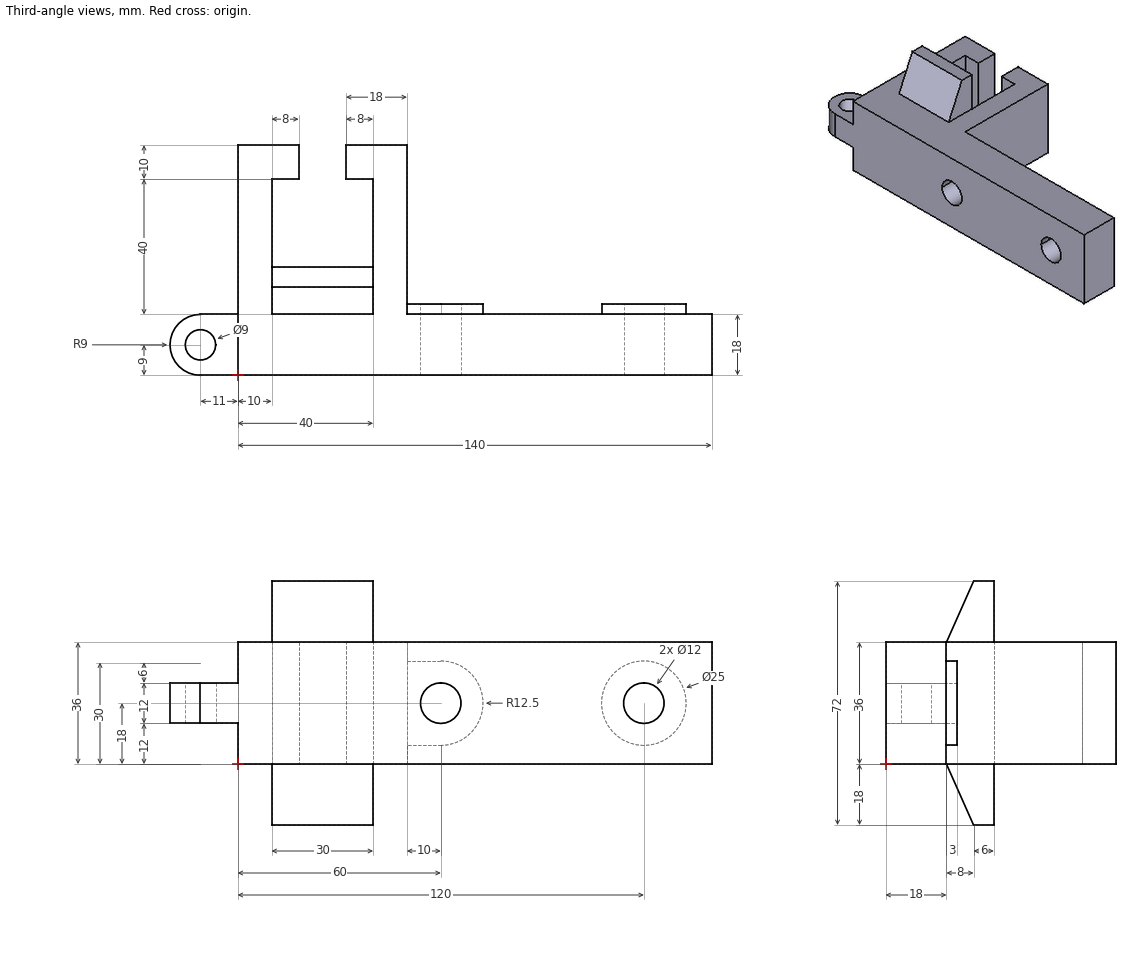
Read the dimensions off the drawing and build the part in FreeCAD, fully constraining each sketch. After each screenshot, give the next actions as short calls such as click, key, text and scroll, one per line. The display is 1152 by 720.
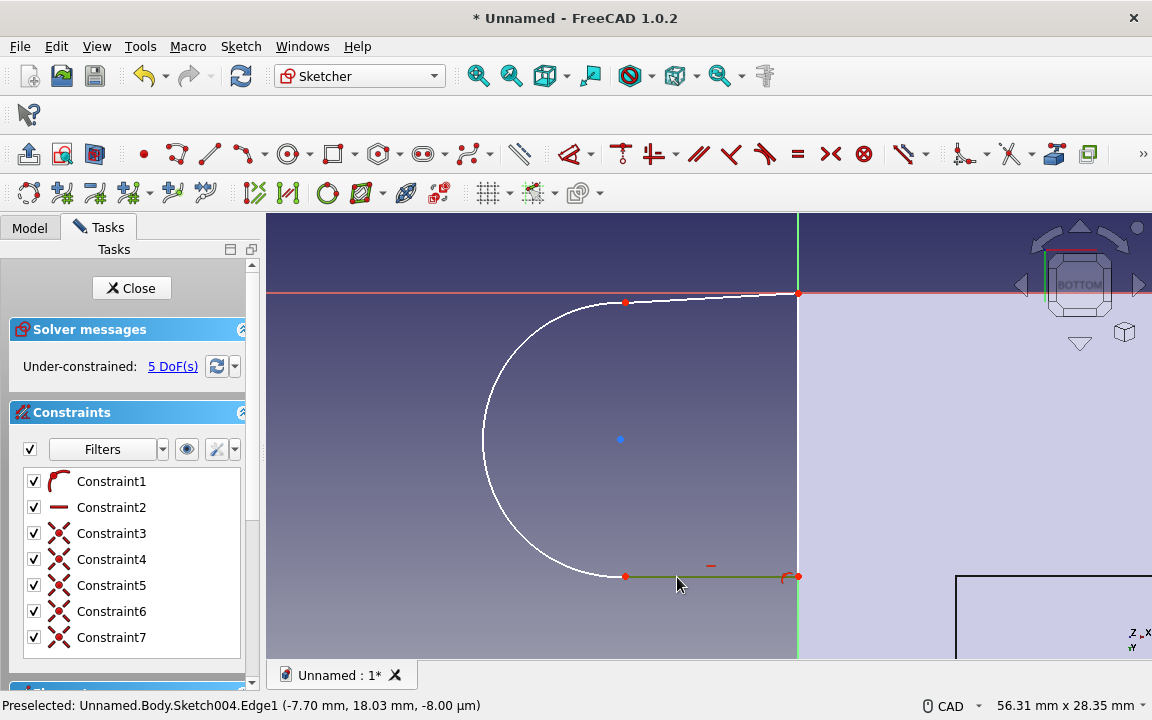
click(510, 358)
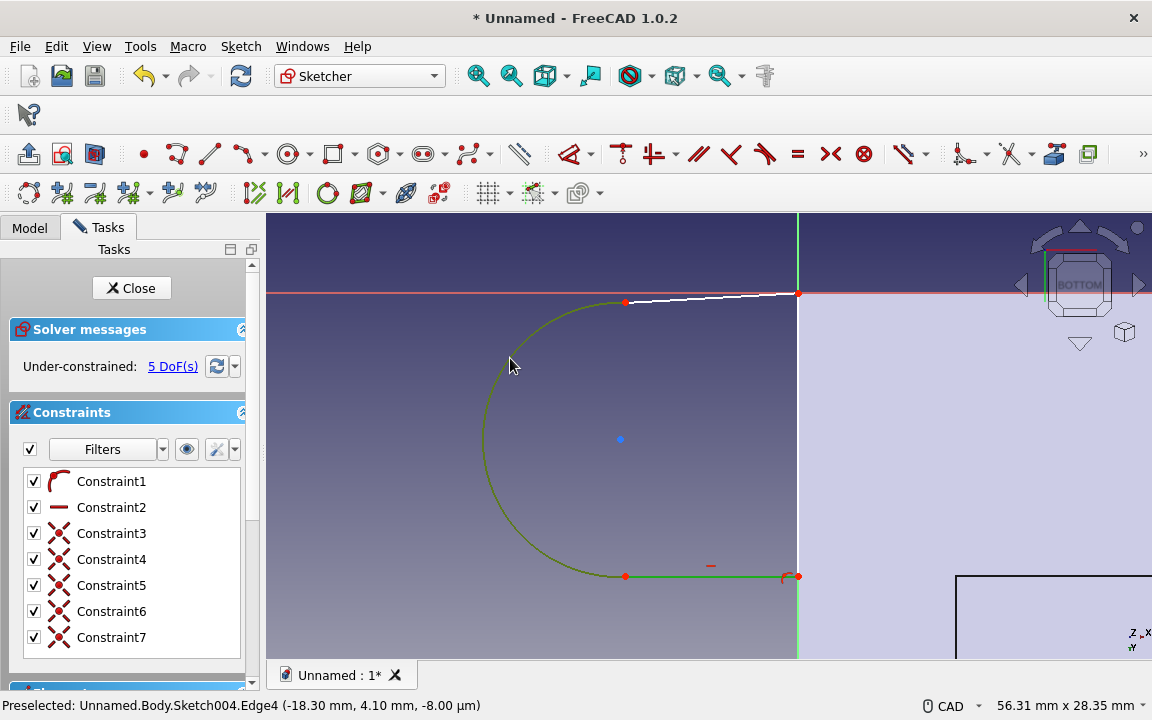
click(765, 154)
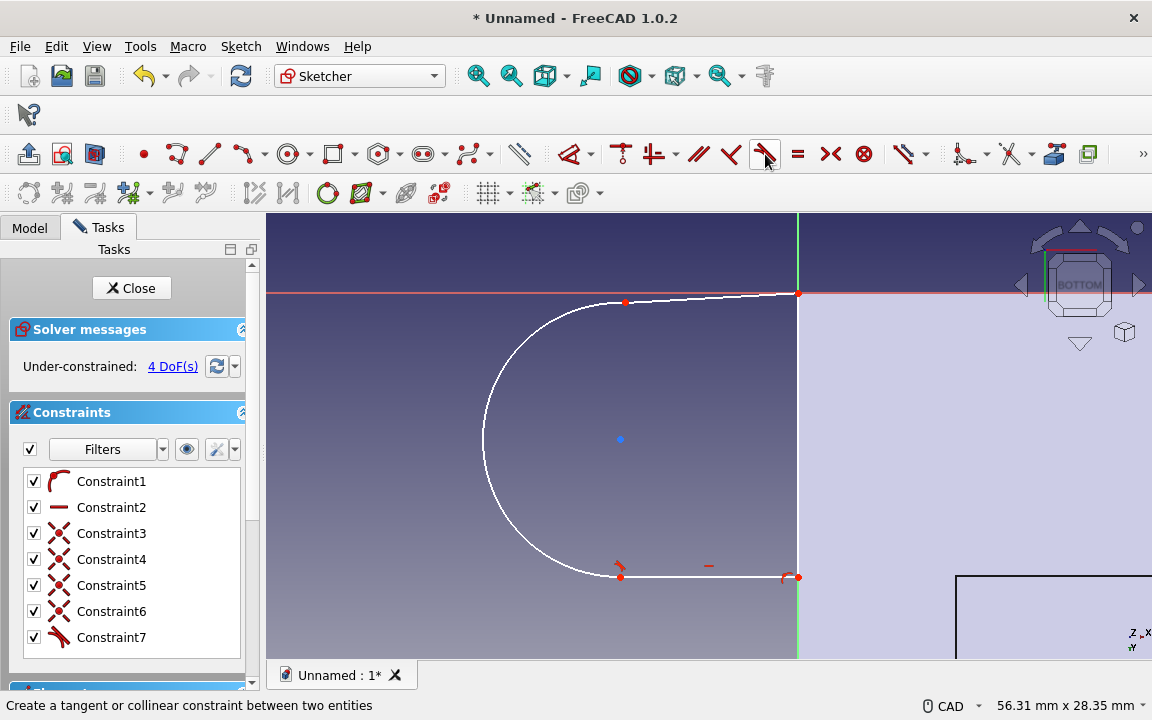
click(746, 296)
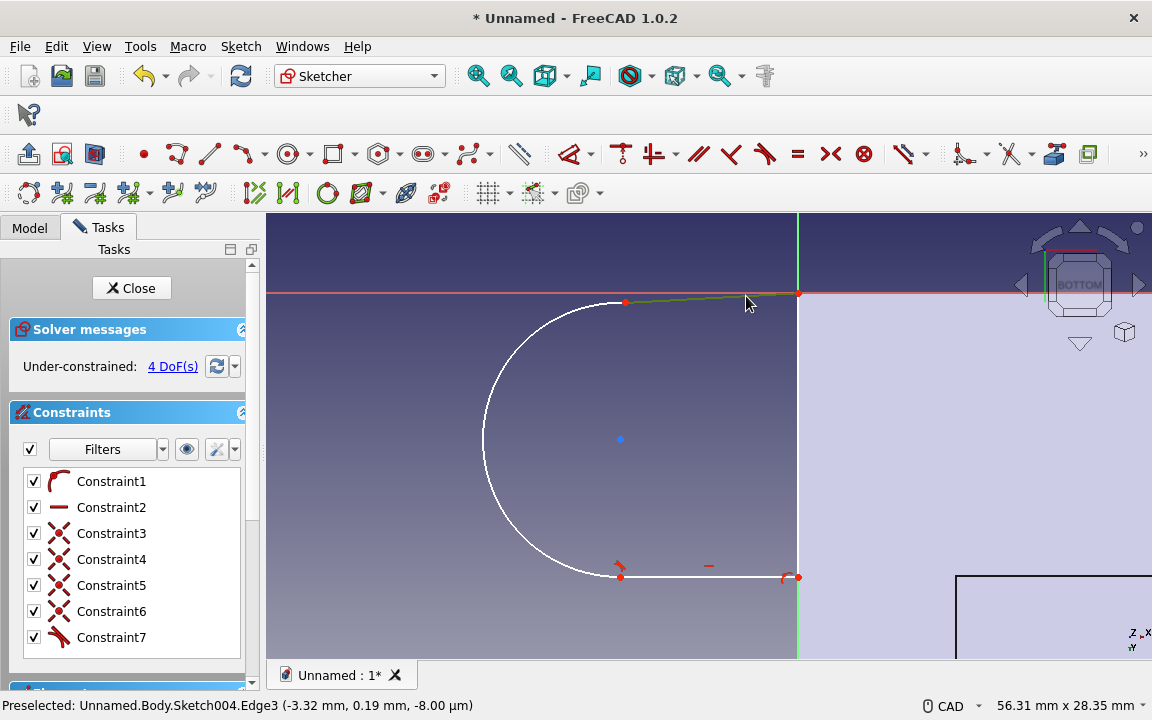
click(511, 357)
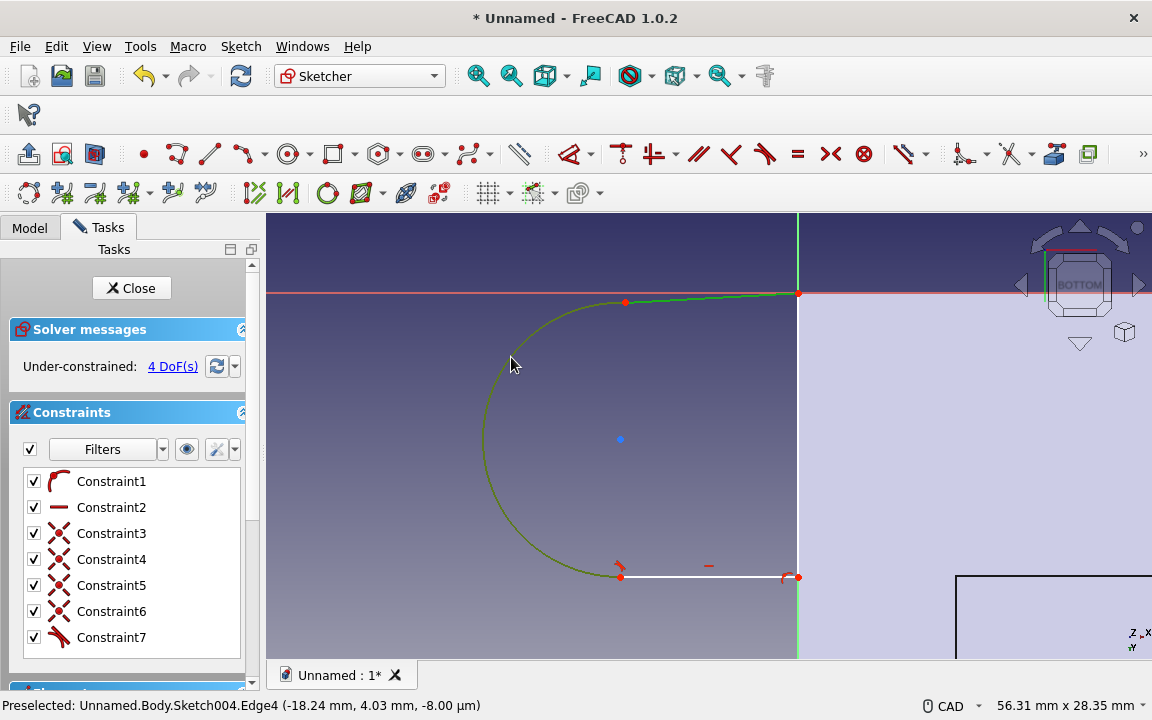
key(t)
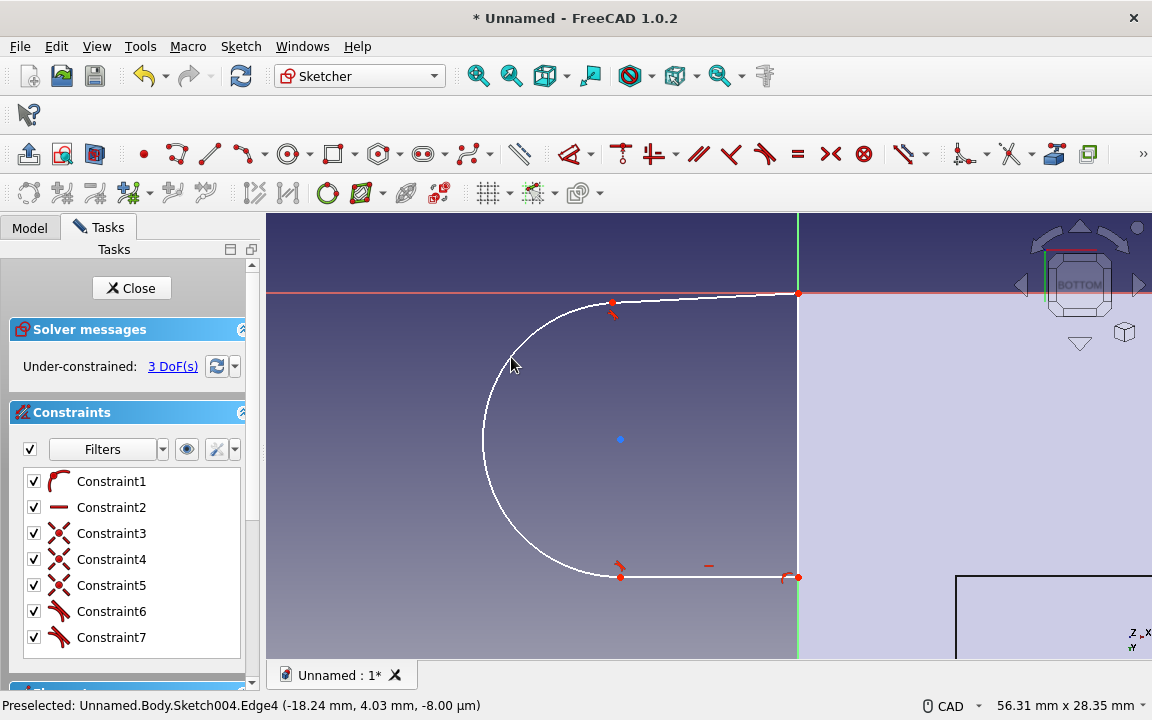
click(743, 296)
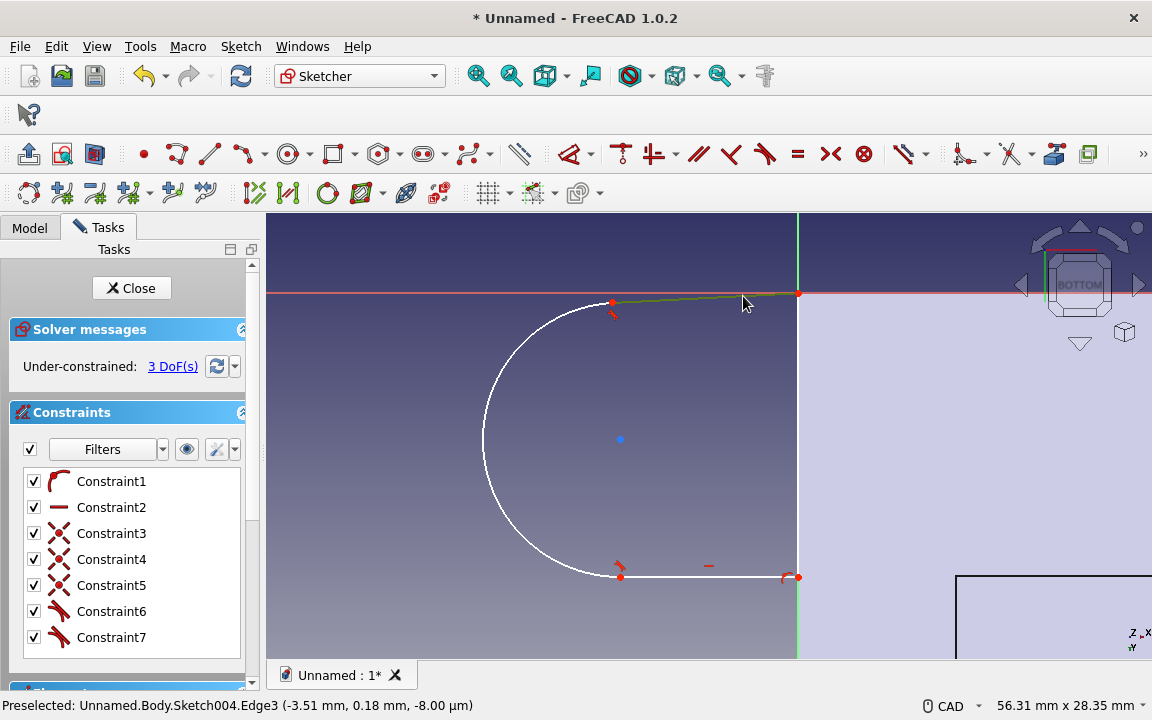
key(h)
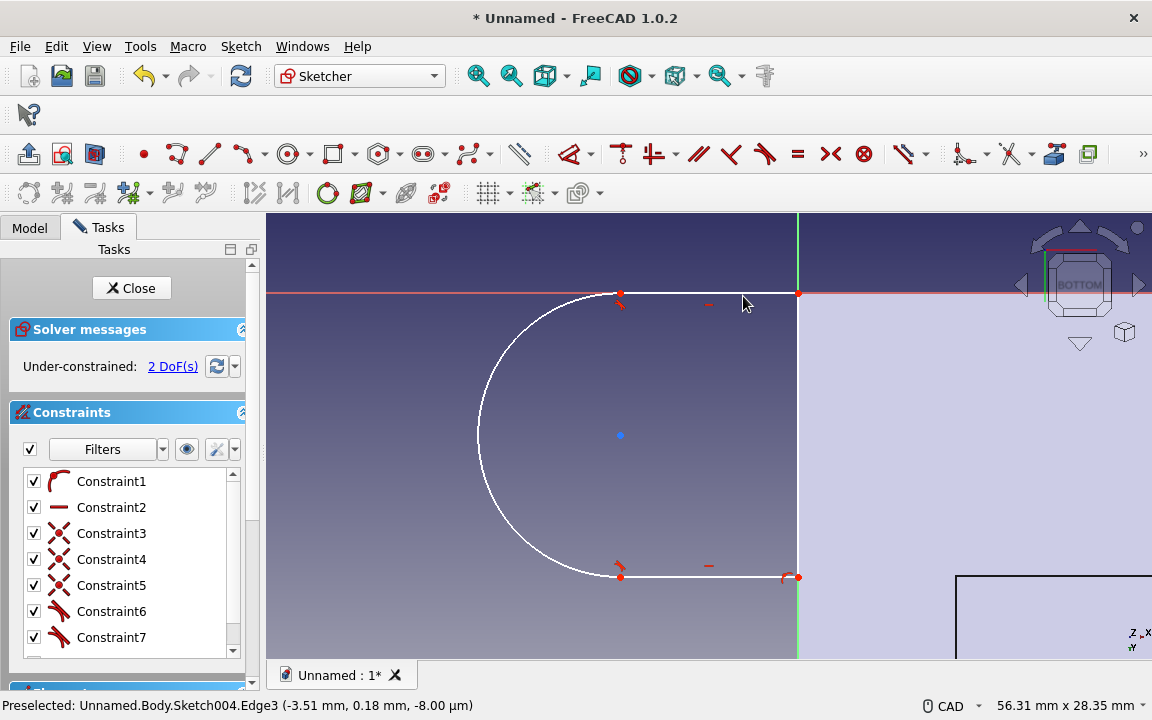
click(568, 154)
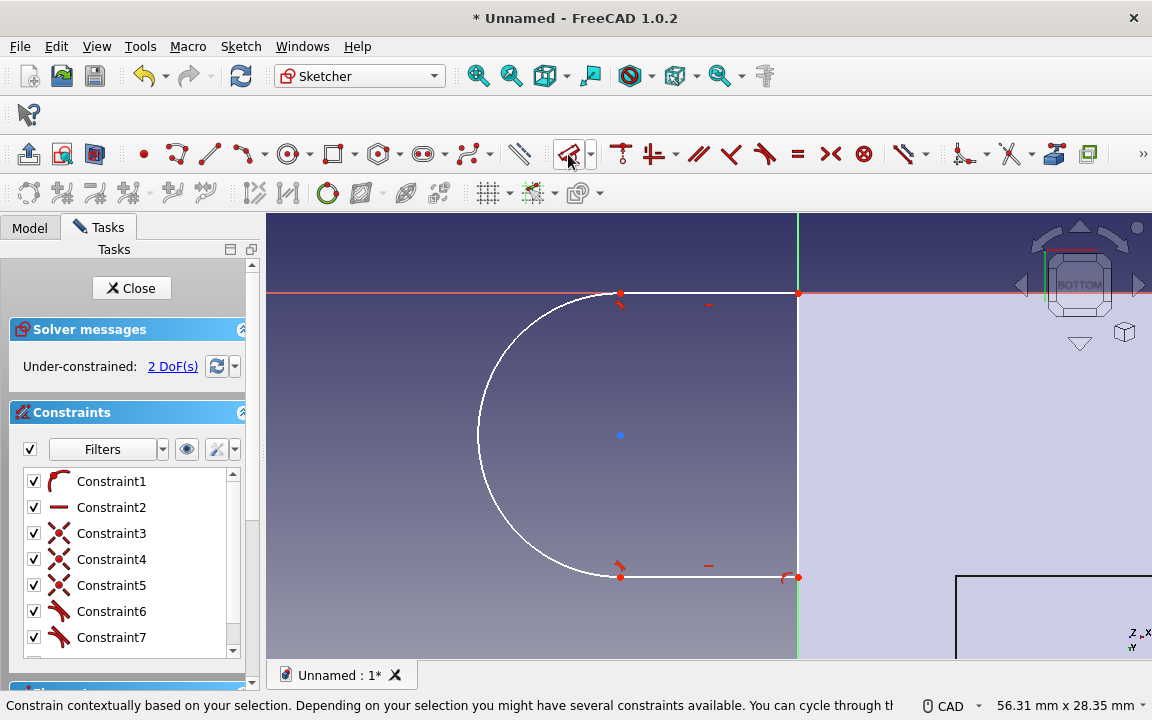
click(505, 352)
click(479, 333)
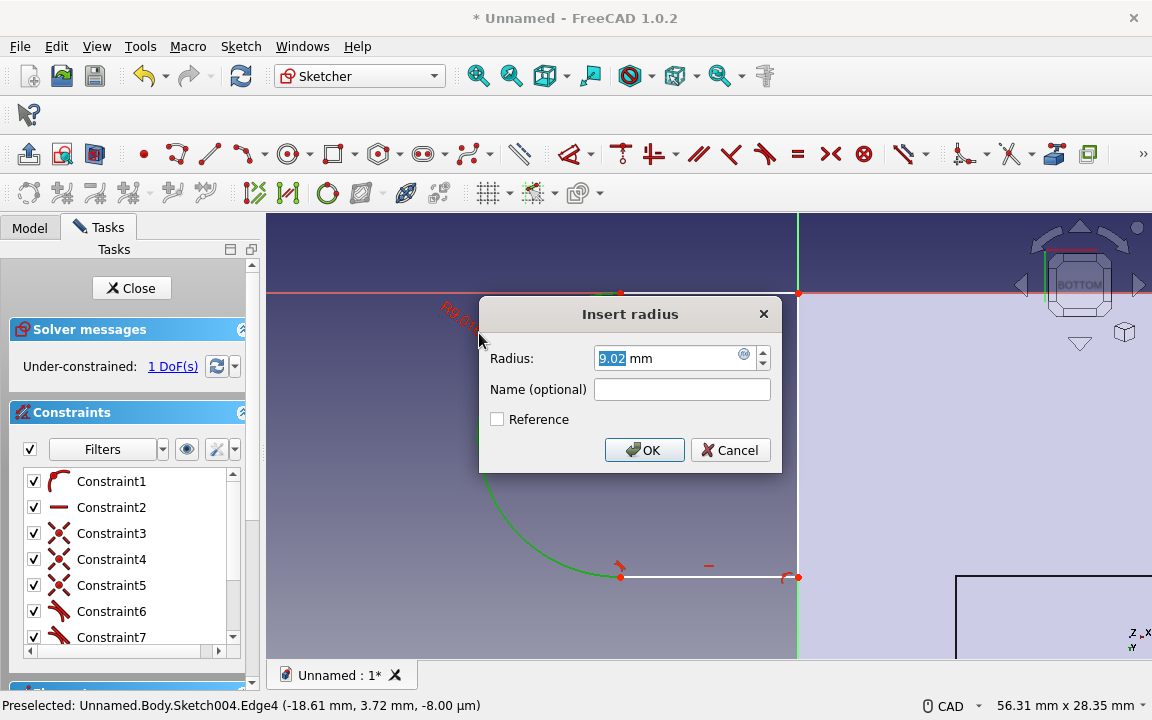
text(9)
key(Return)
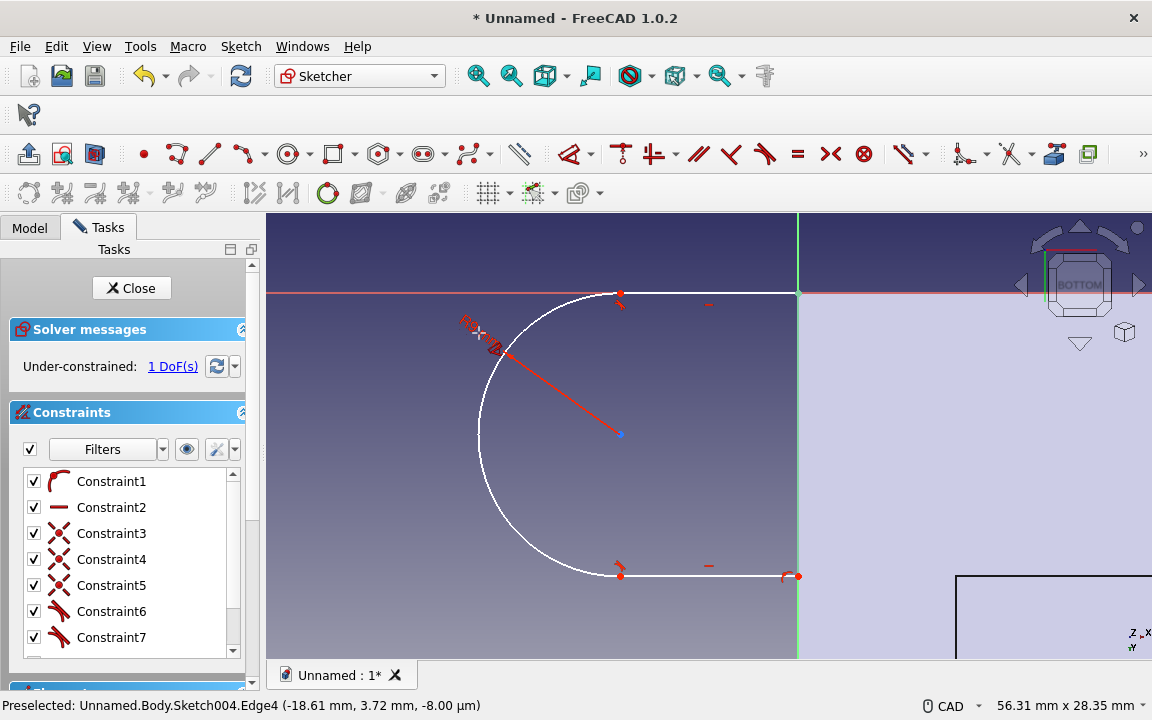
click(674, 576)
click(709, 610)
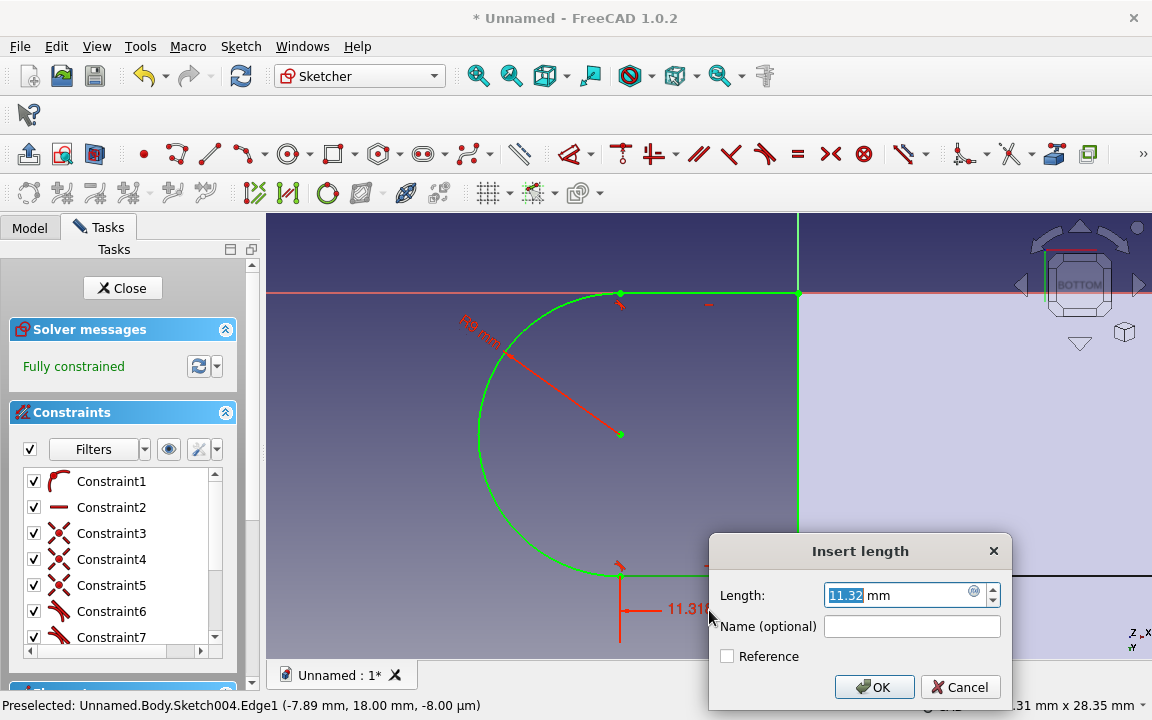
text(11)
key(Return)
key(Escape)